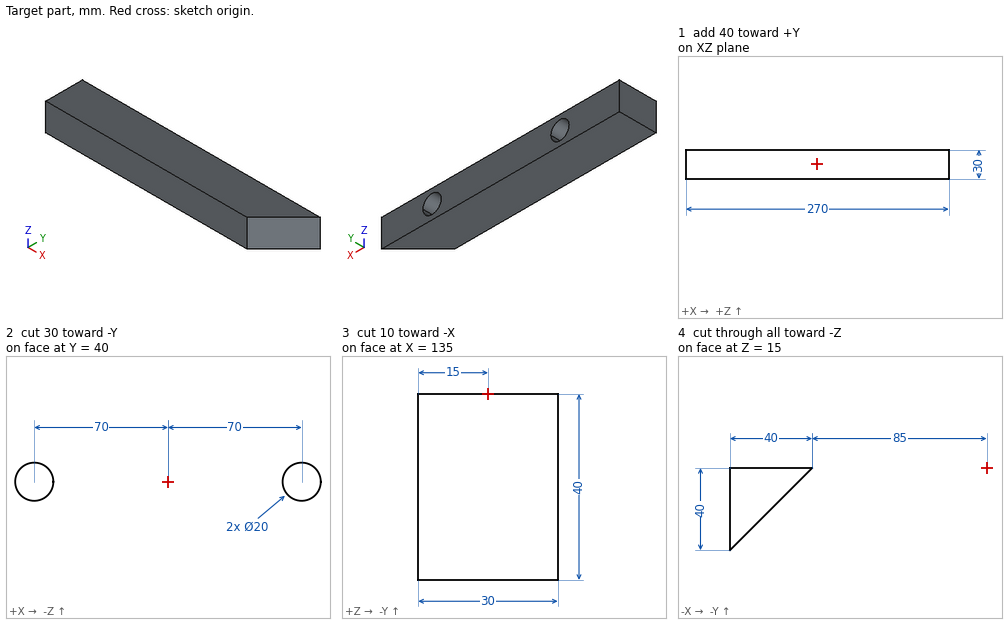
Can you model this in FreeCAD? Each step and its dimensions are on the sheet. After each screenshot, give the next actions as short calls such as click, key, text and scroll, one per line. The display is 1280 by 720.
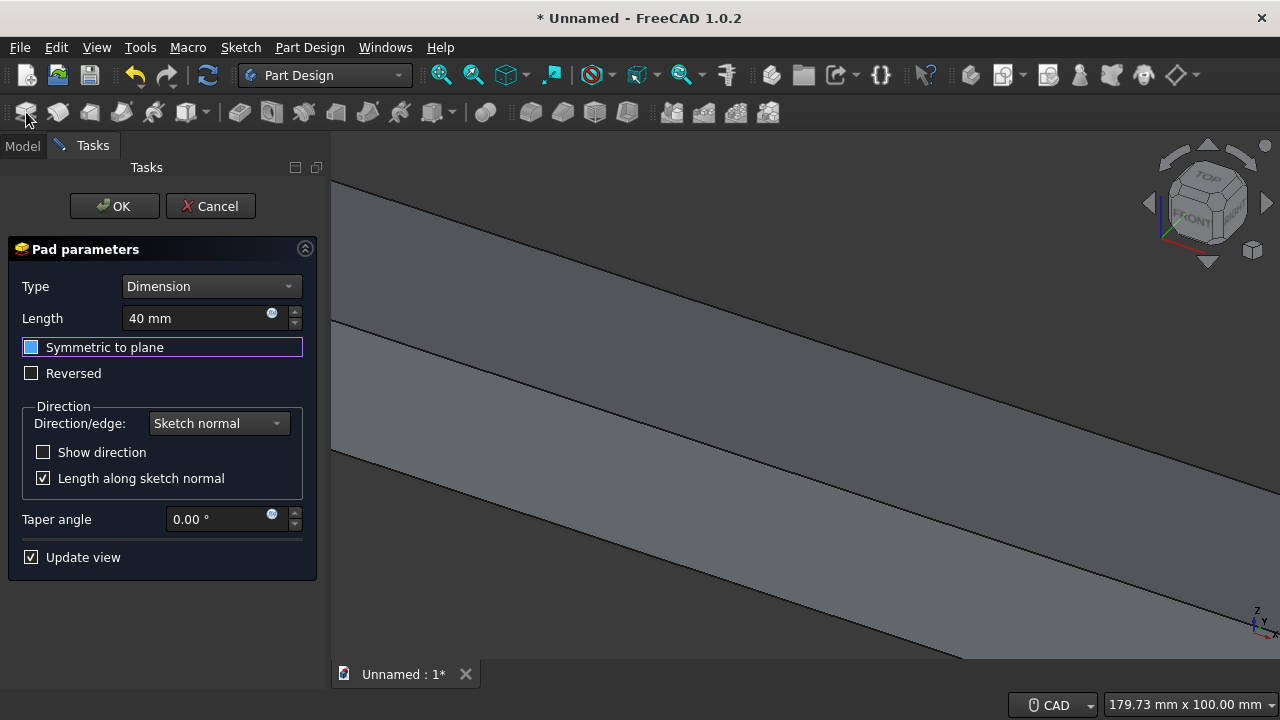
click(30, 373)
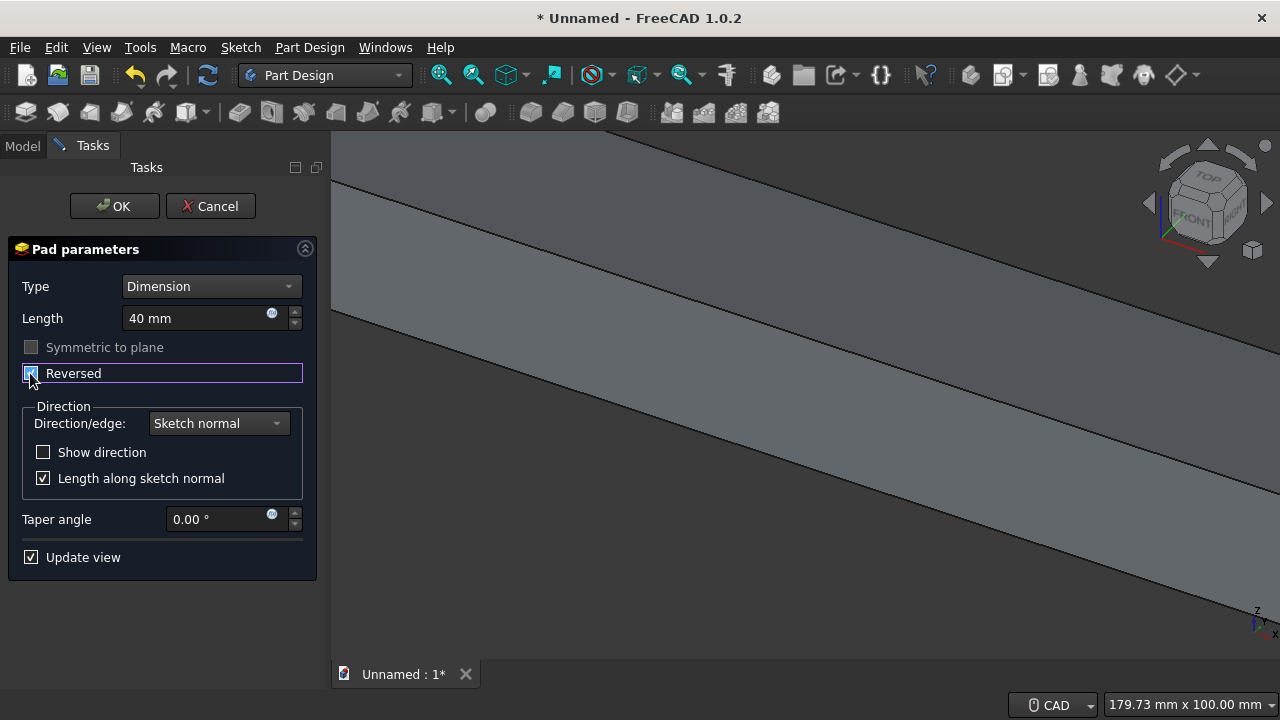
click(115, 206)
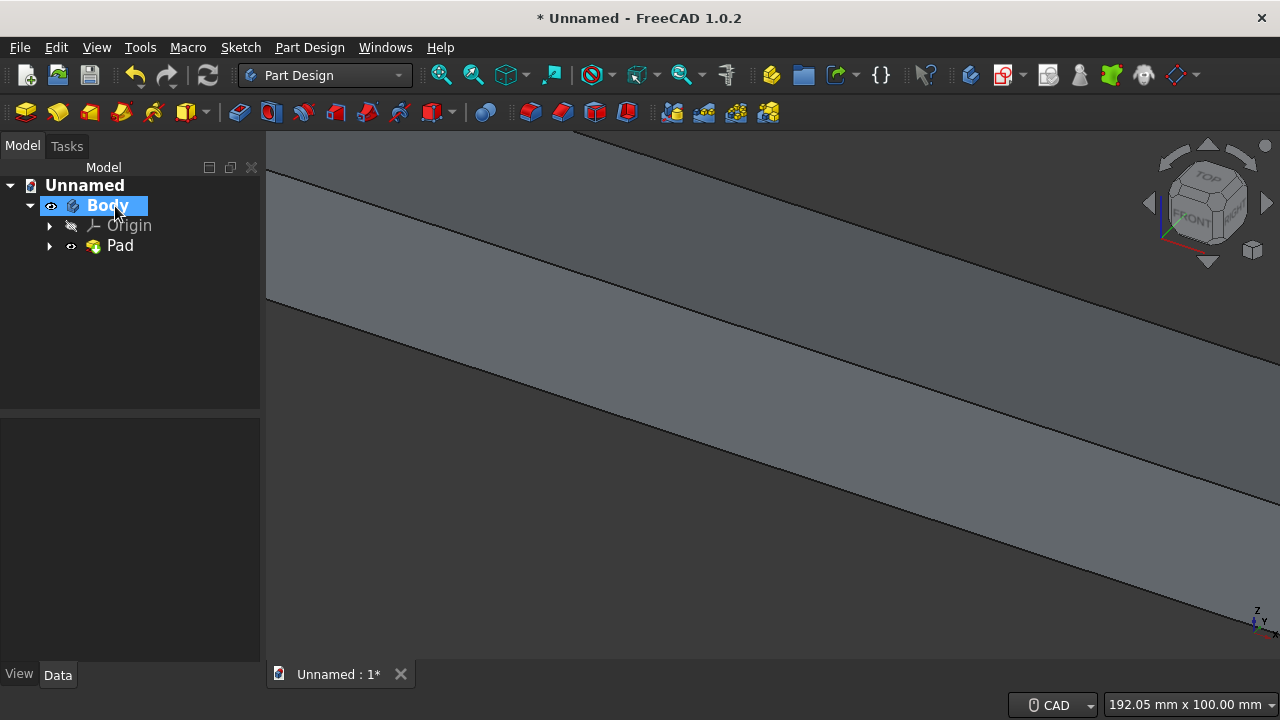
click(442, 76)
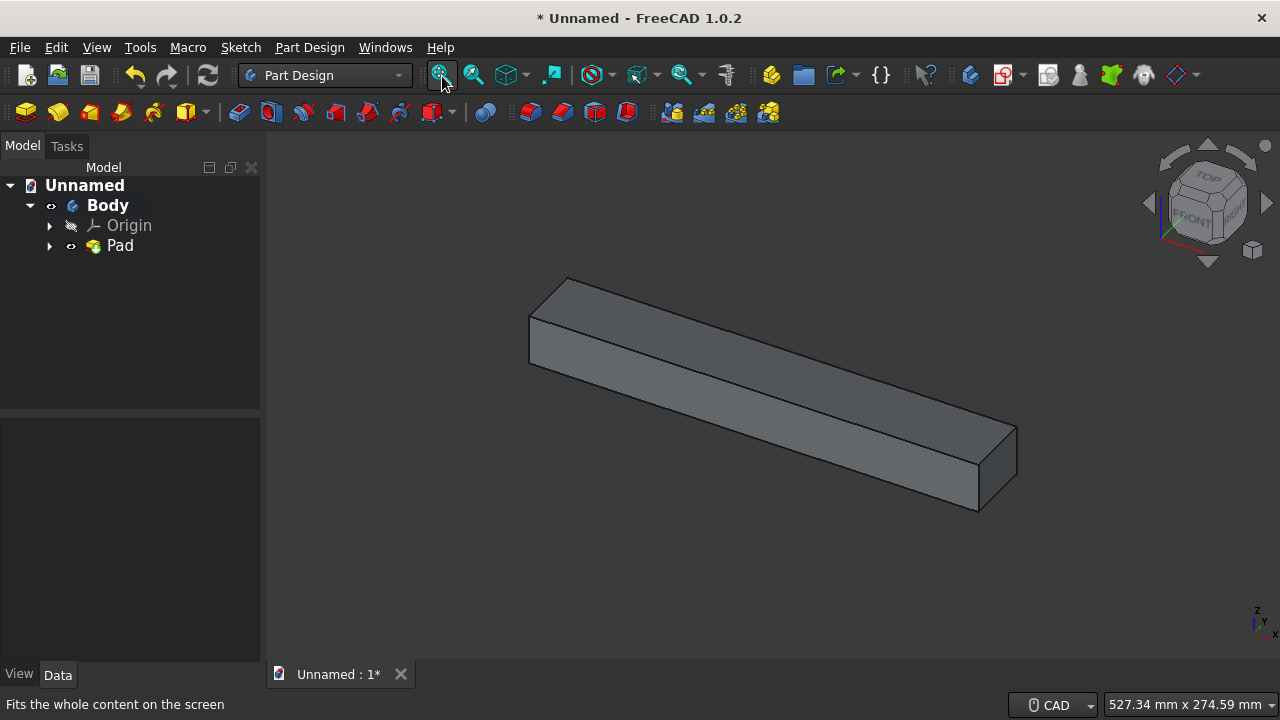
key(4)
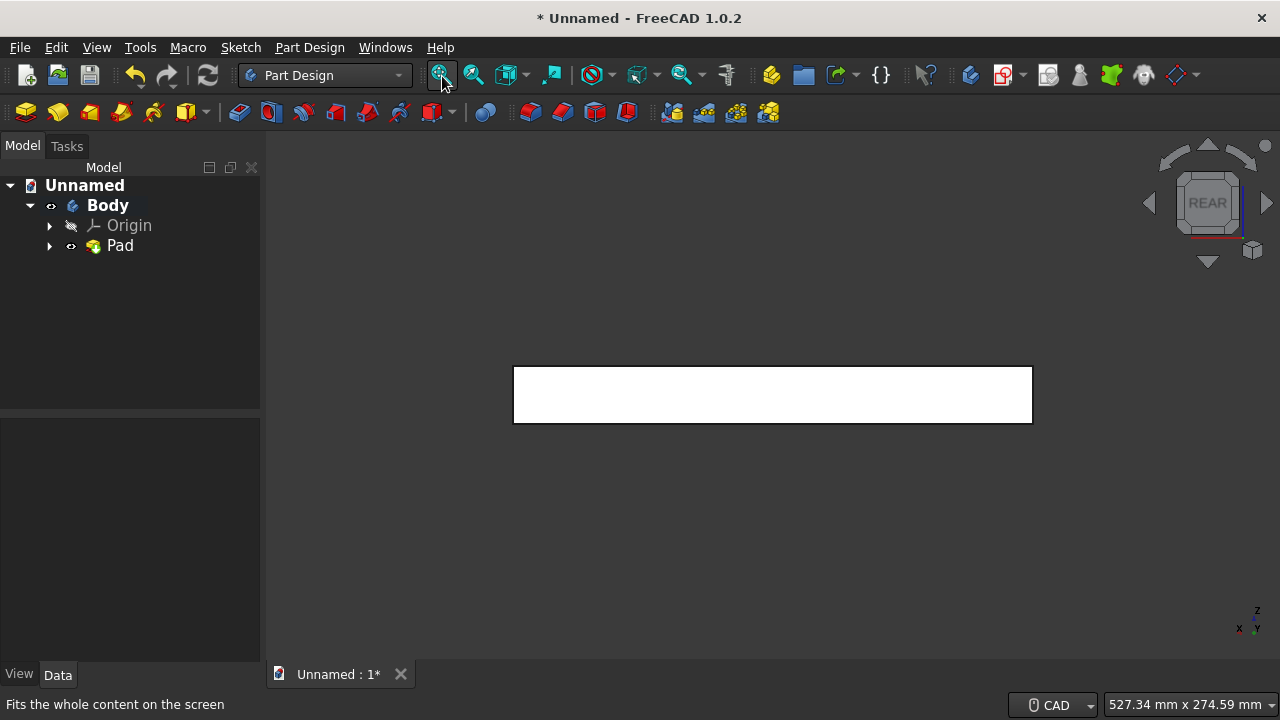
click(550, 394)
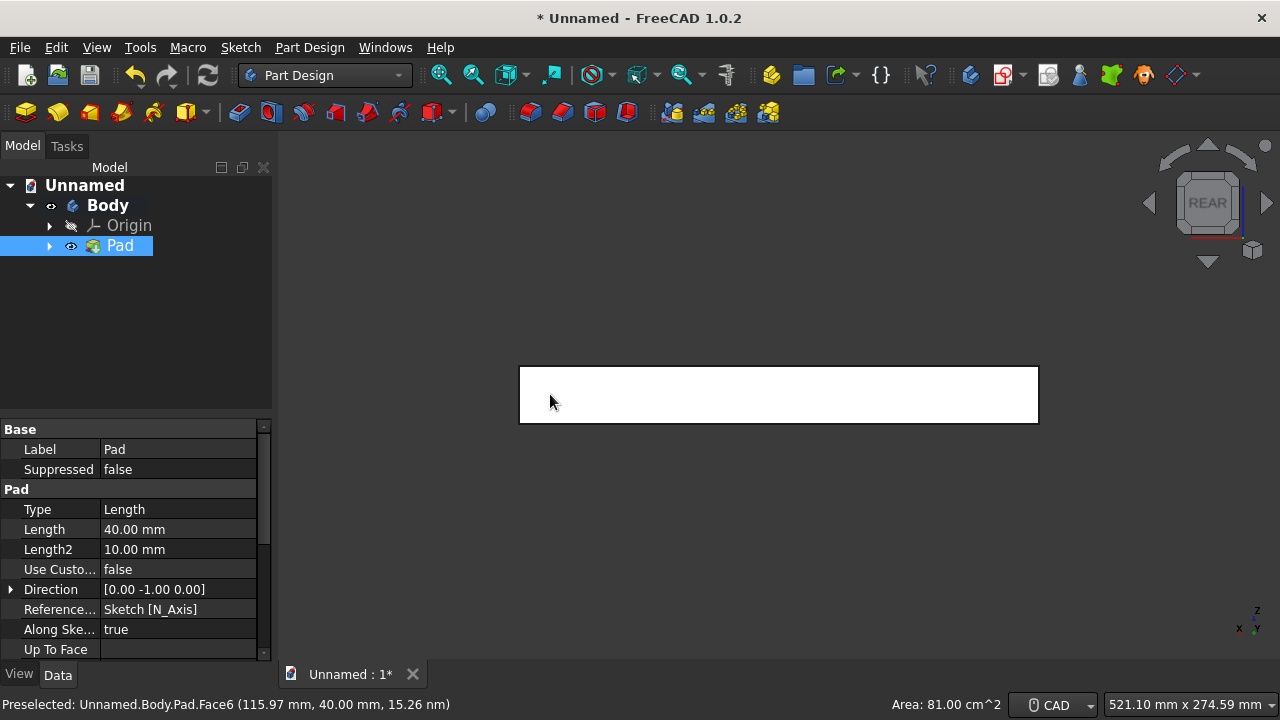
click(1004, 76)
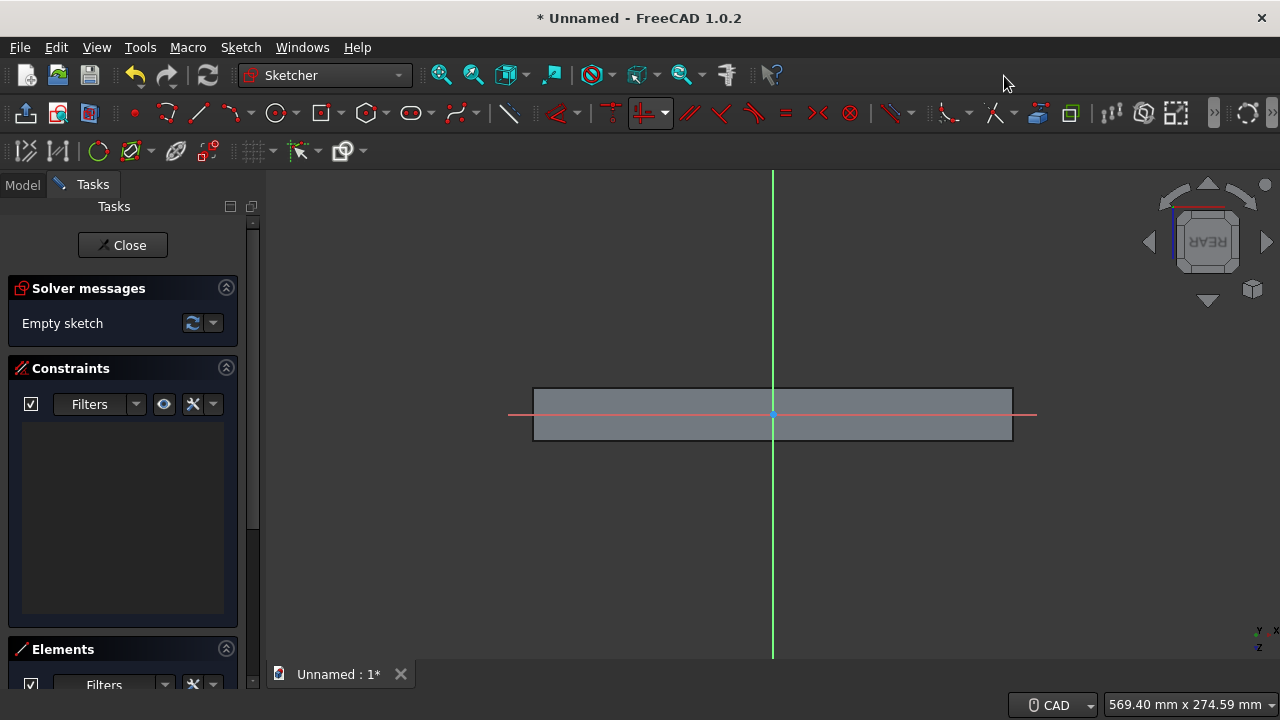
scroll(829, 414, up, 4)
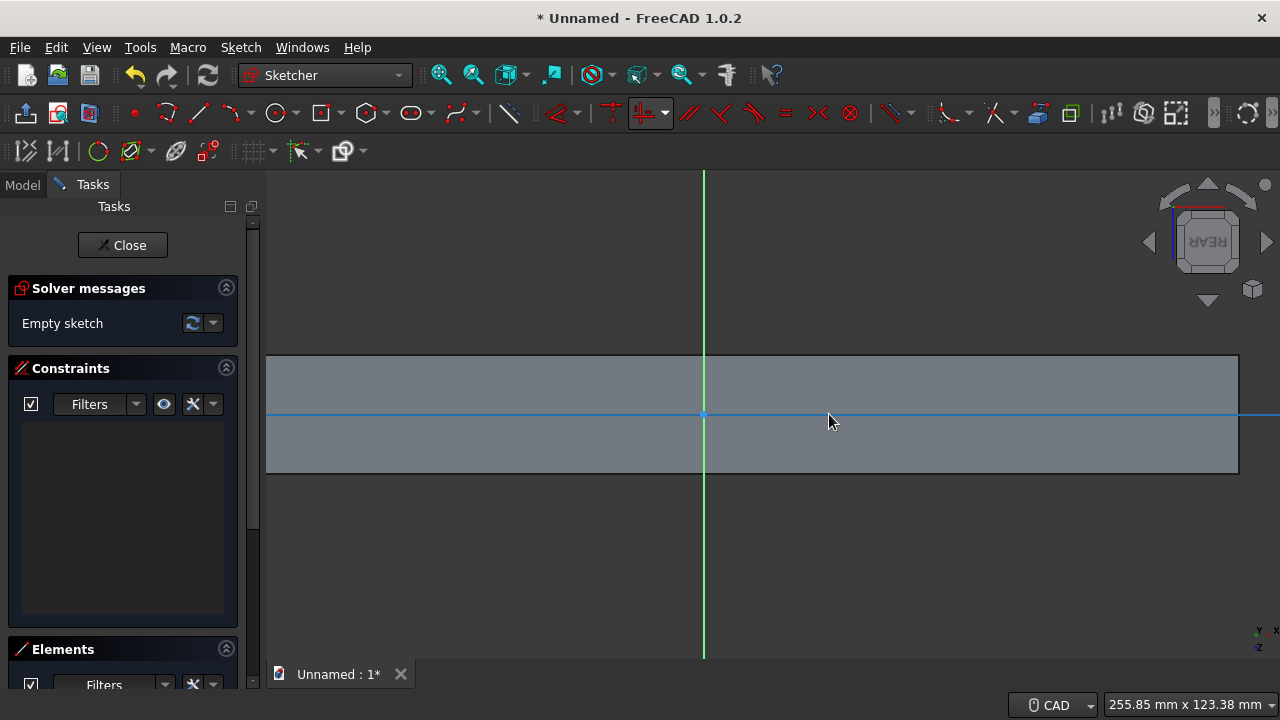
click(276, 114)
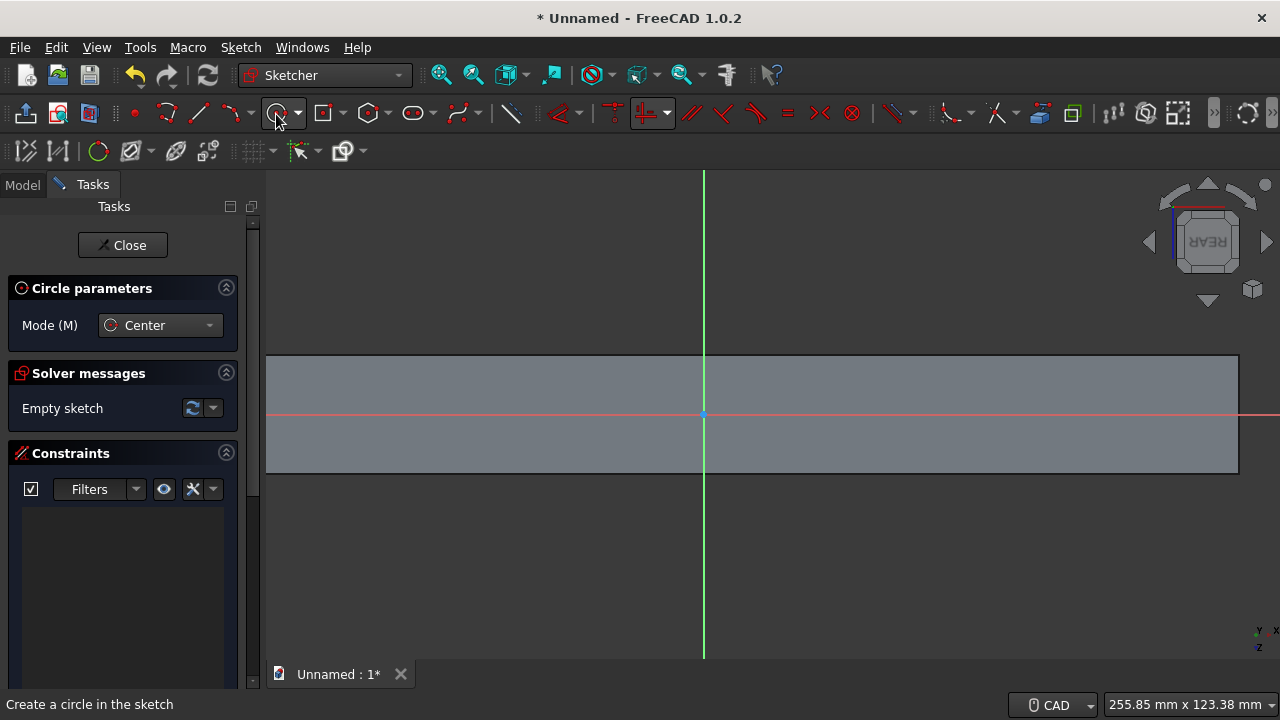
click(981, 414)
move(1009, 386)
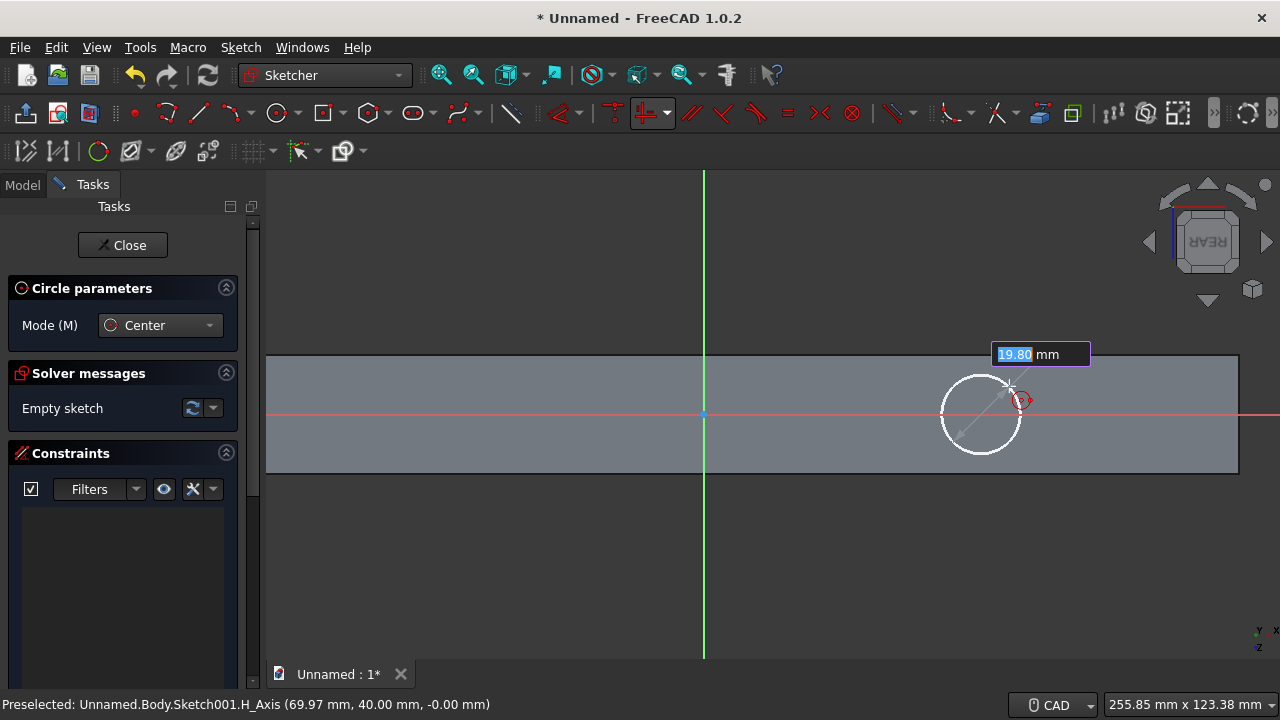
text(20)
key(Return)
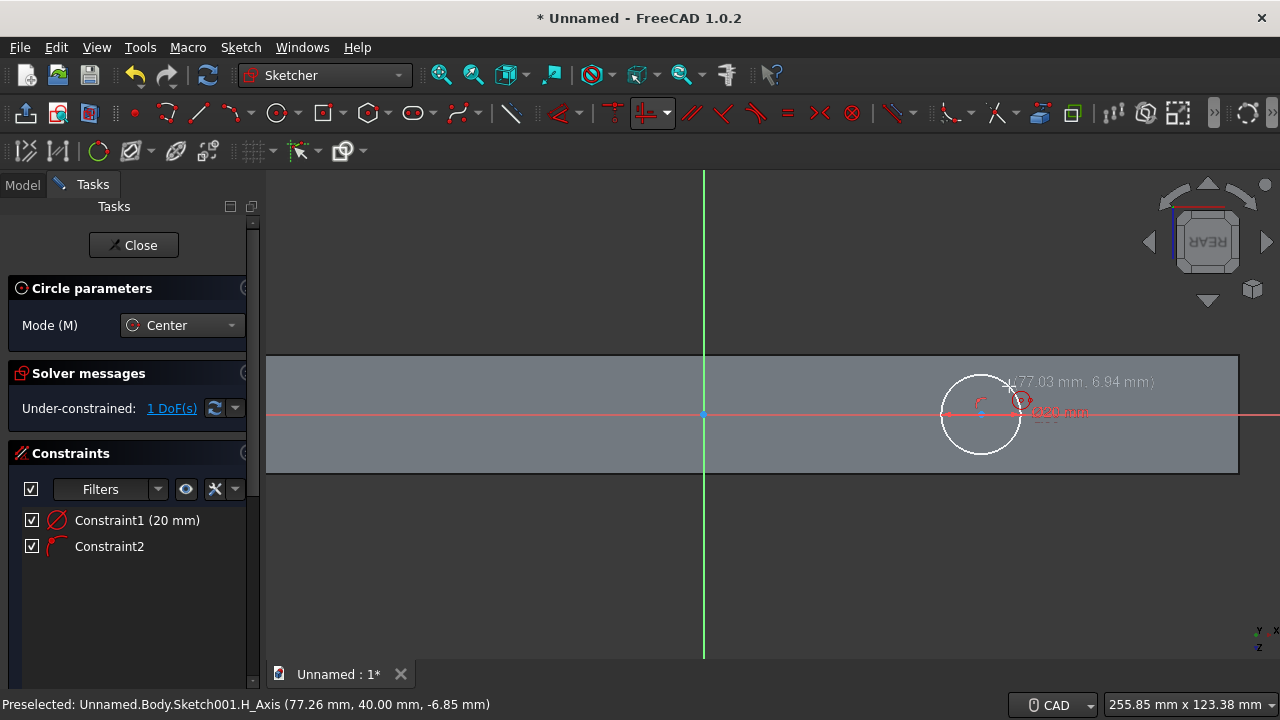
click(426, 414)
move(454, 386)